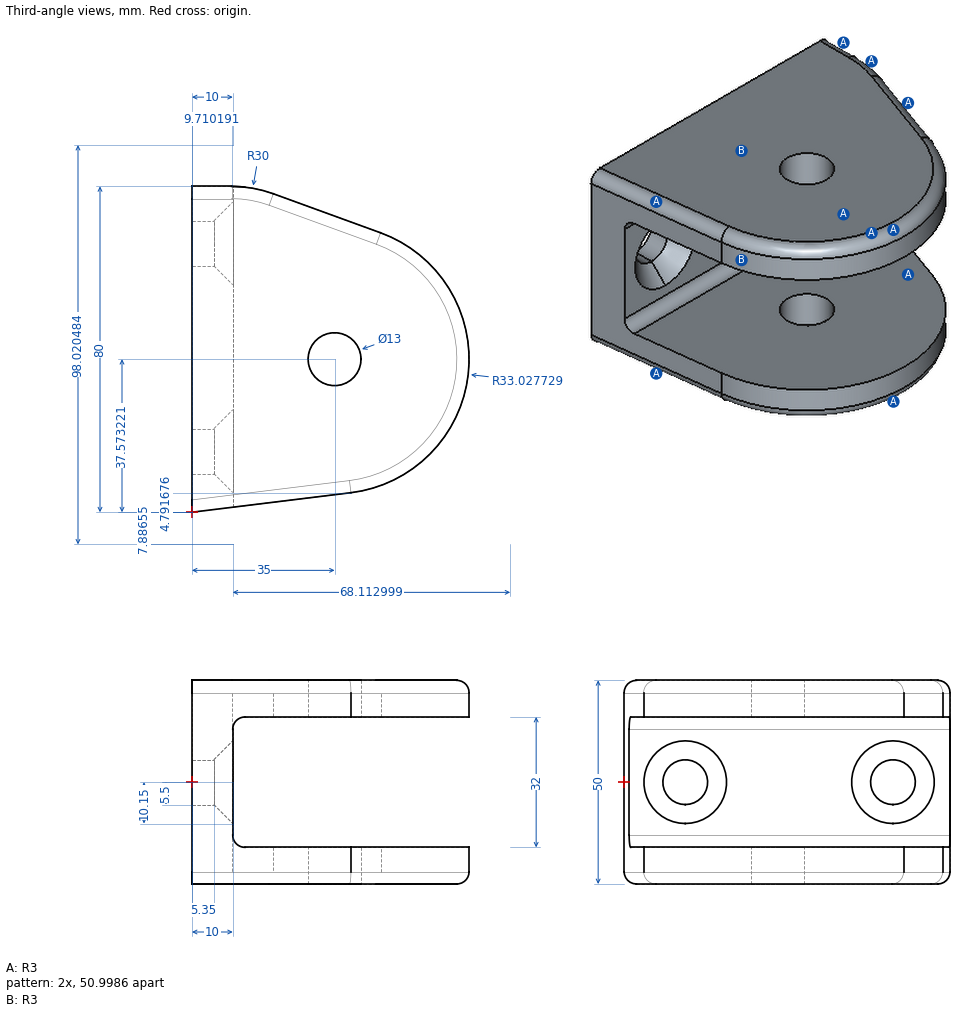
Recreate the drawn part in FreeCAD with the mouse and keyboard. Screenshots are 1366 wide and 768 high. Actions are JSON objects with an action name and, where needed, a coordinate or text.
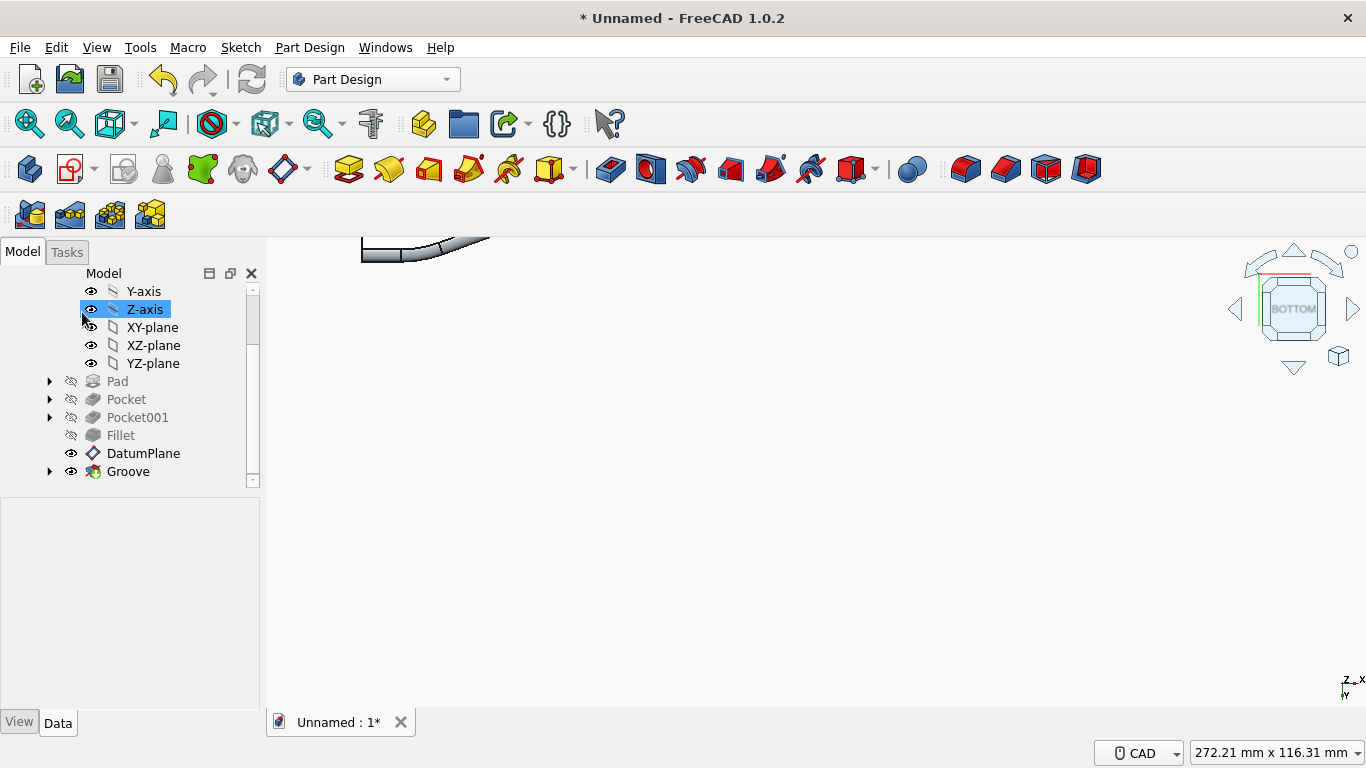
{"action": "left_click", "coordinate": [116, 453]}
{"action": "key", "text": "space"}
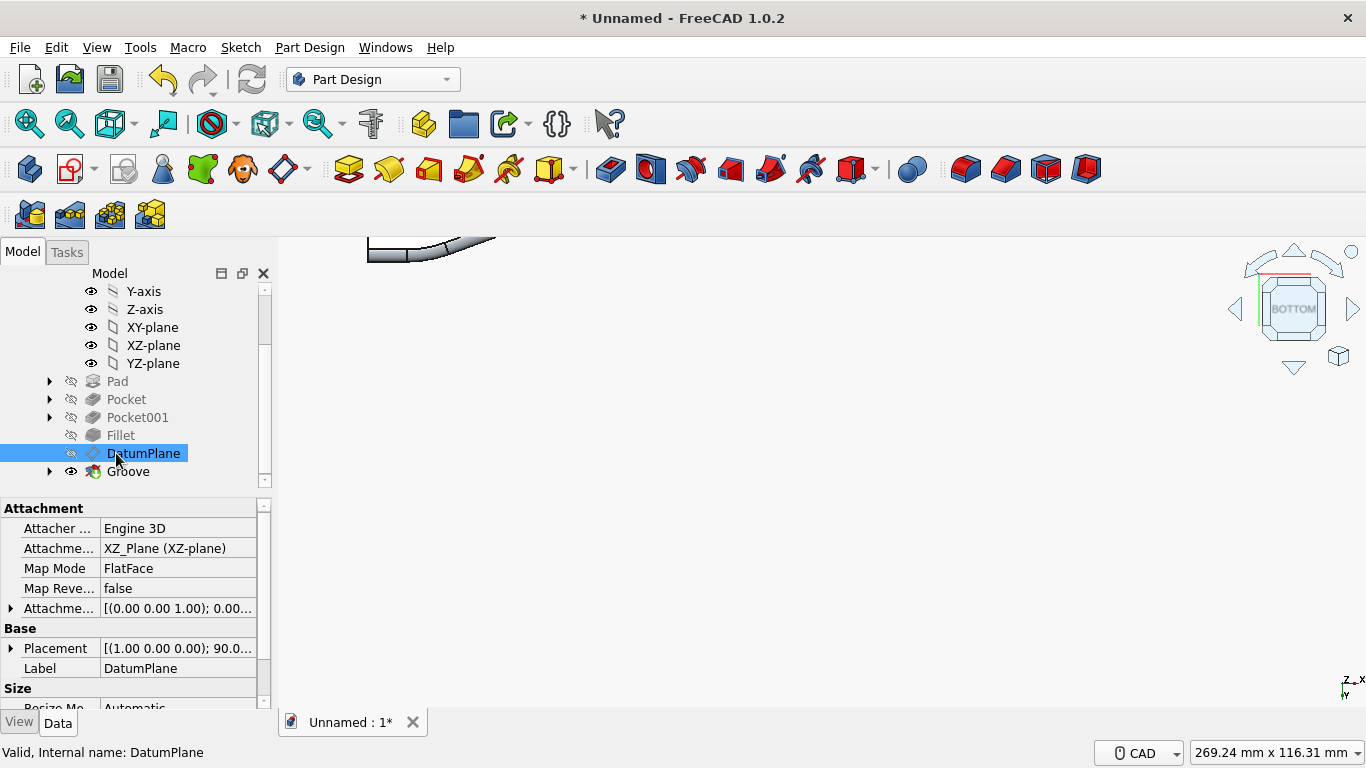
{"action": "left_click", "coordinate": [30, 124]}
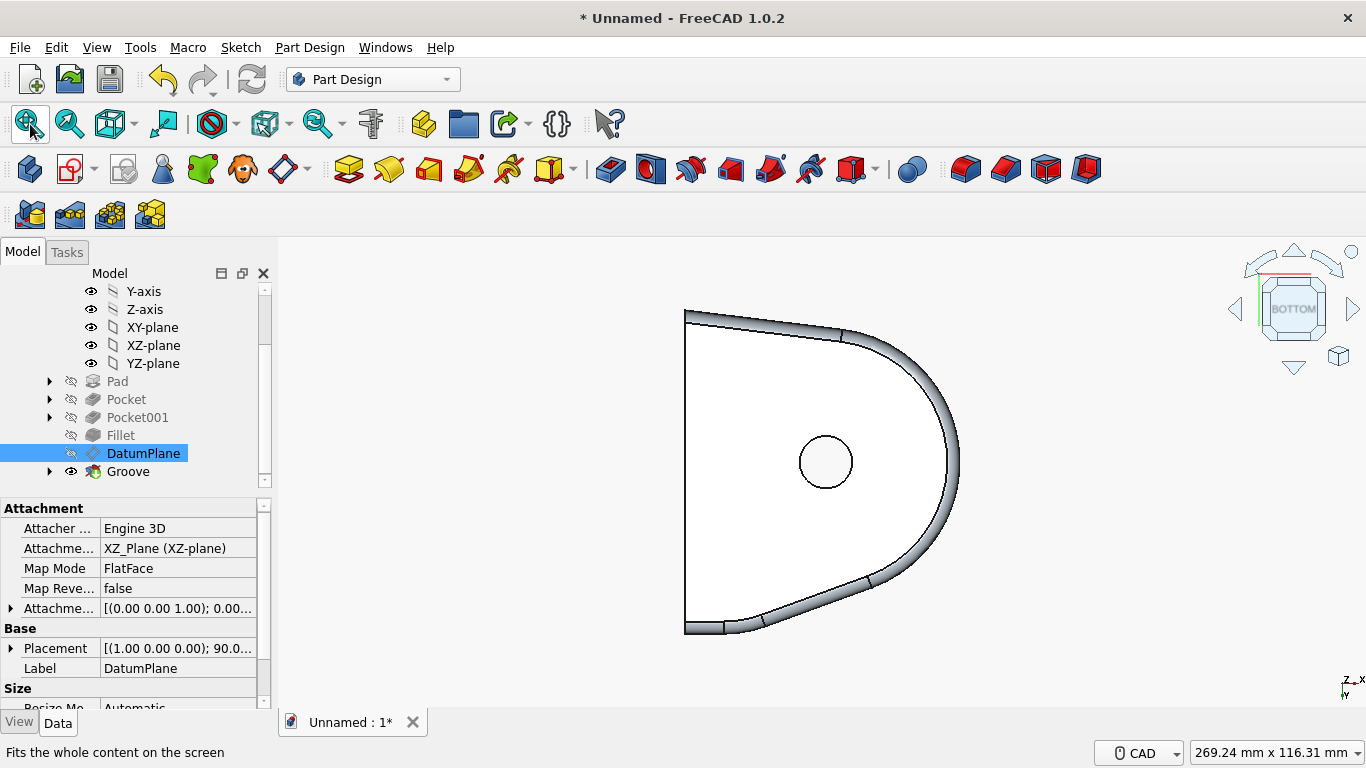
{"action": "left_click", "coordinate": [116, 471]}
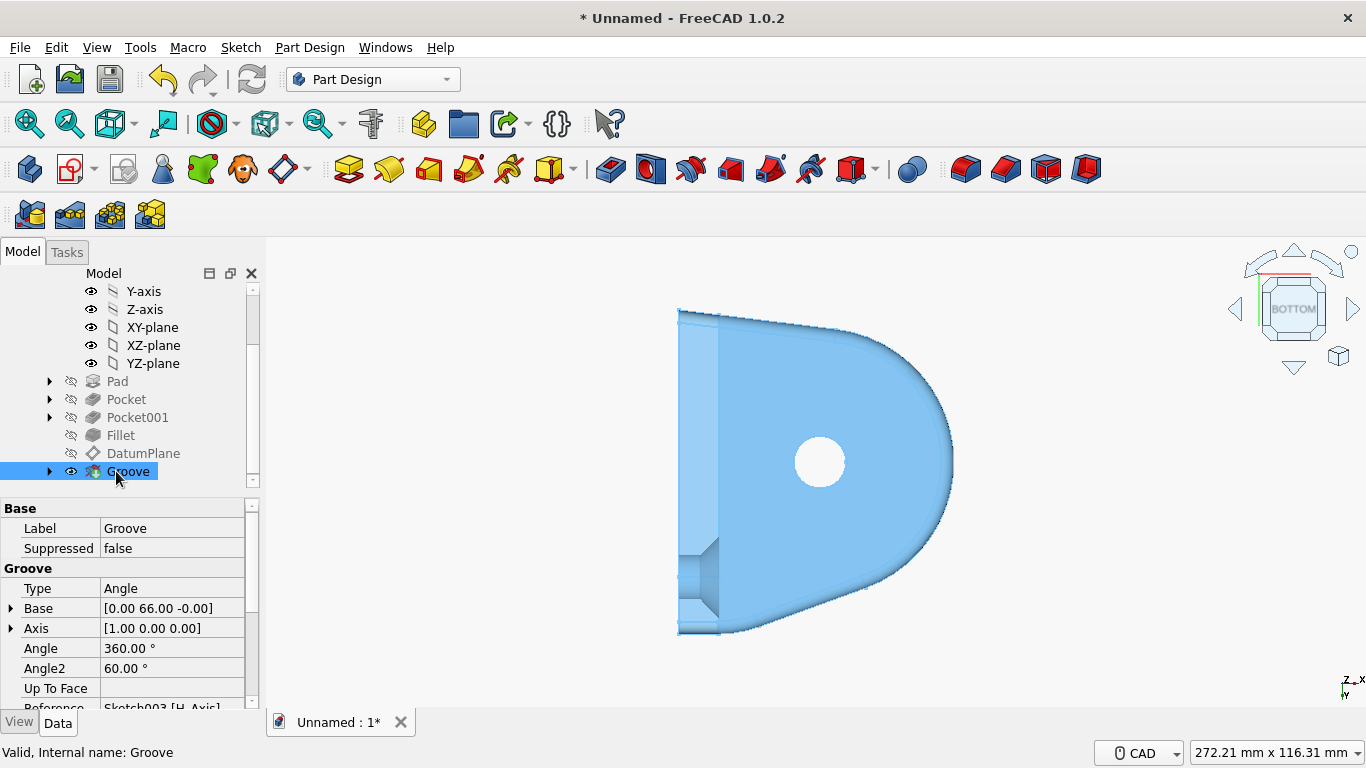
{"action": "left_click", "coordinate": [70, 214]}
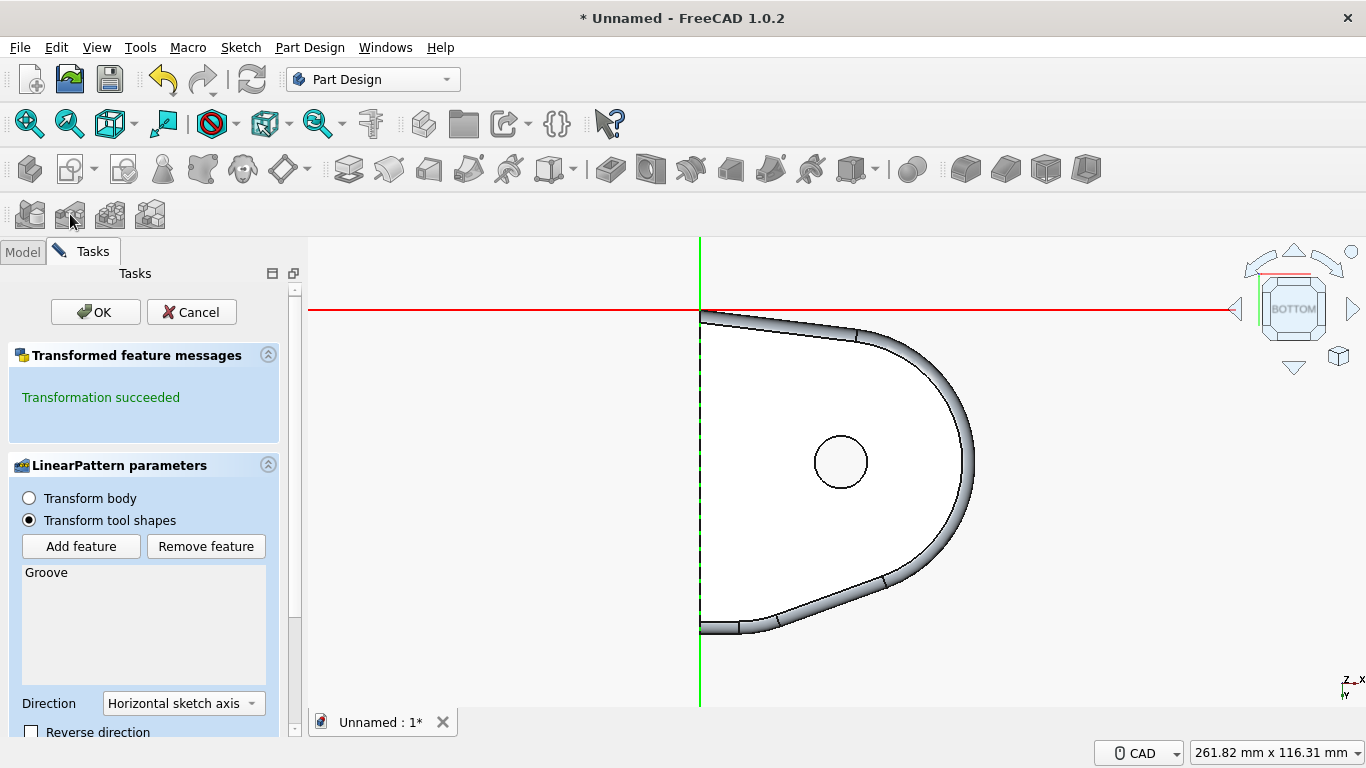
{"action": "left_click", "coordinate": [184, 704]}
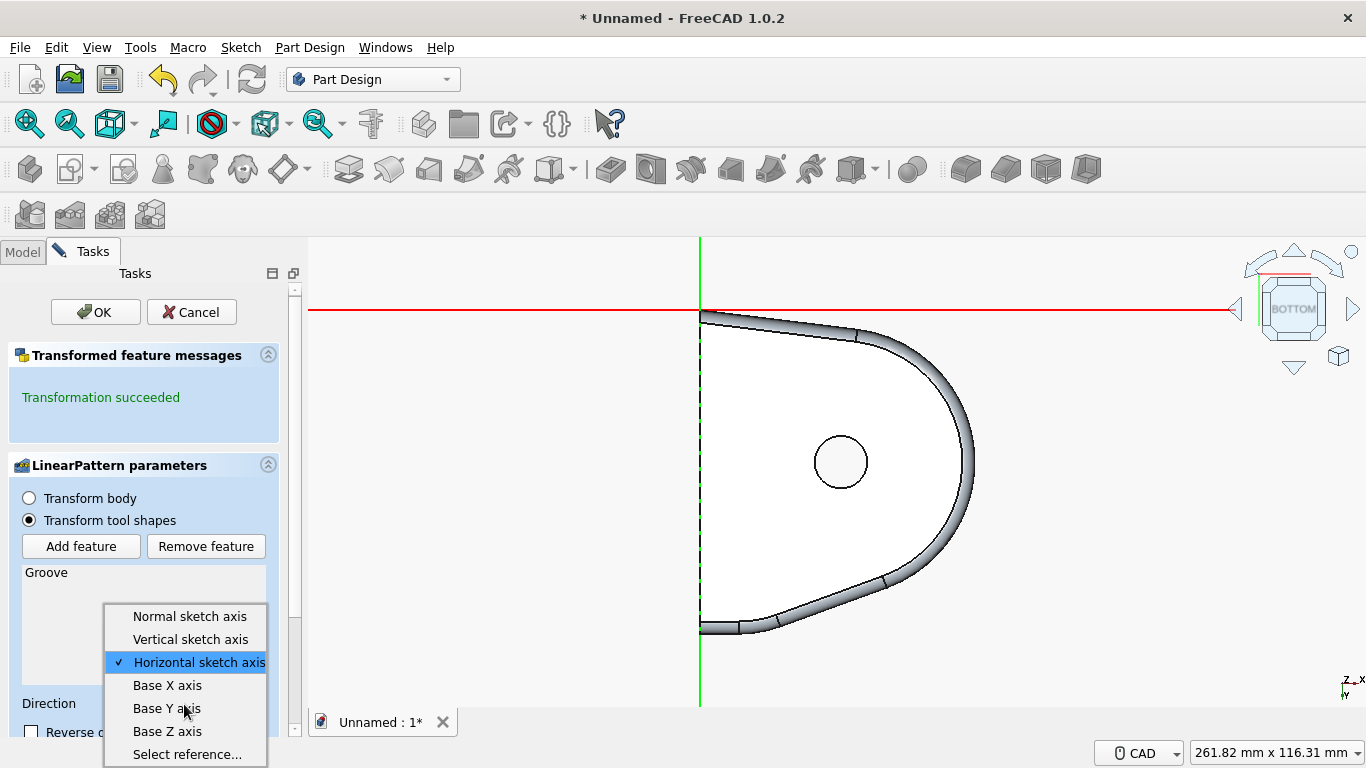
{"action": "left_click", "coordinate": [184, 708]}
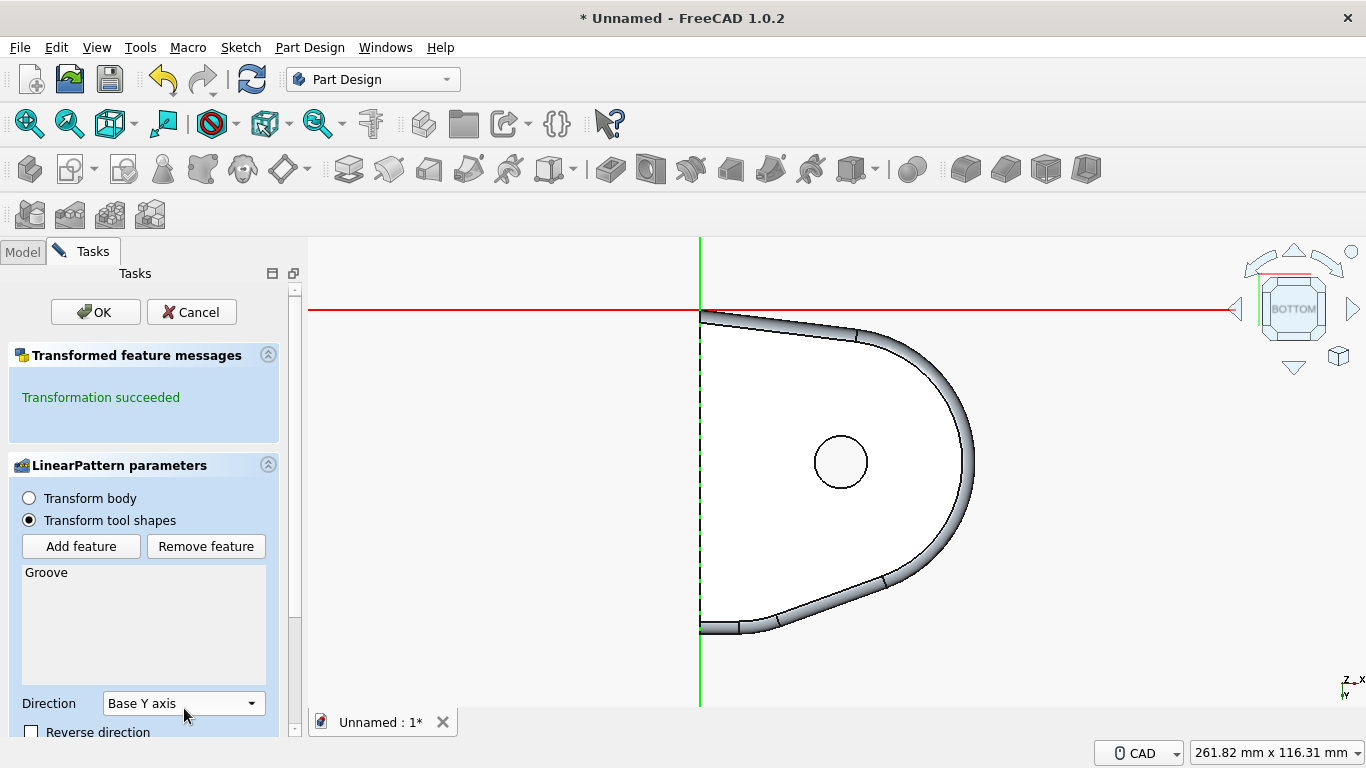
{"action": "scroll", "coordinate": [295, 510], "scroll_direction": "down", "scroll_amount": 2}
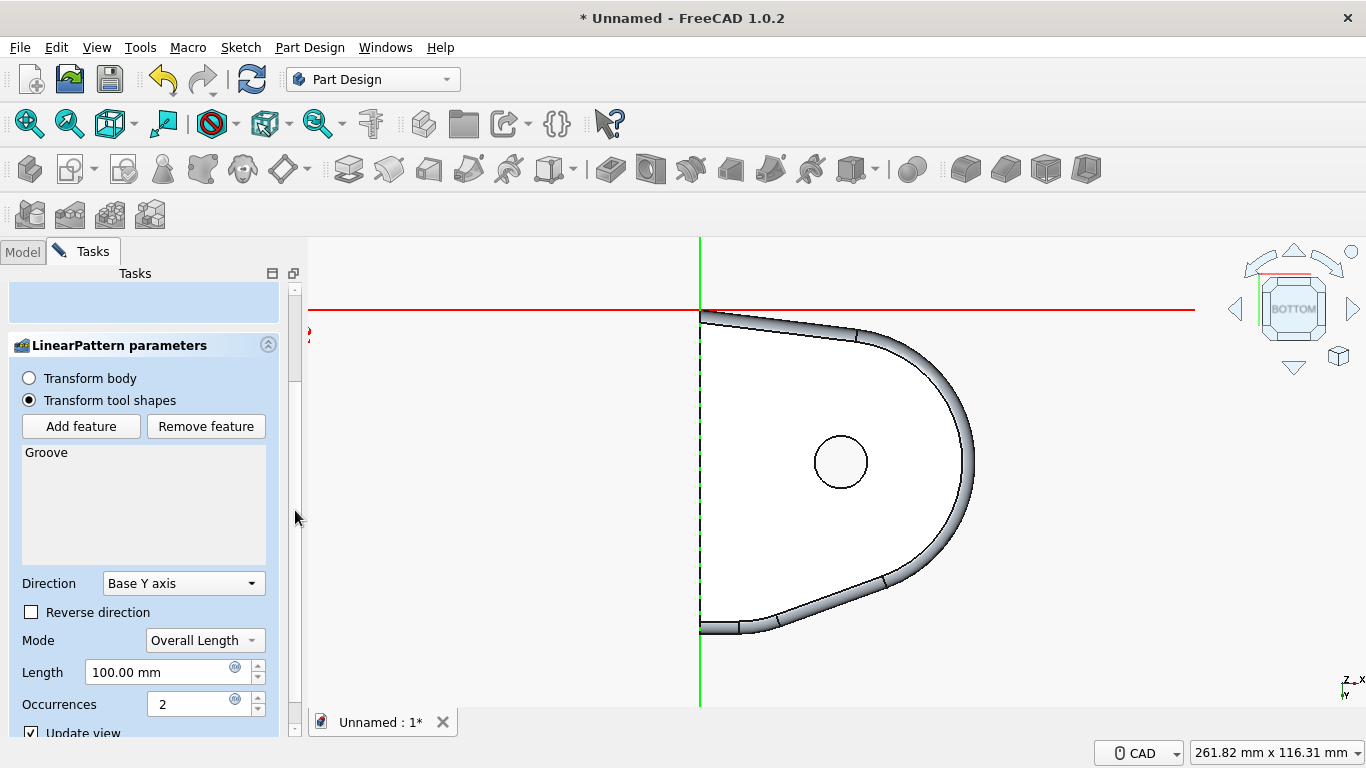
{"action": "left_click", "coordinate": [206, 640]}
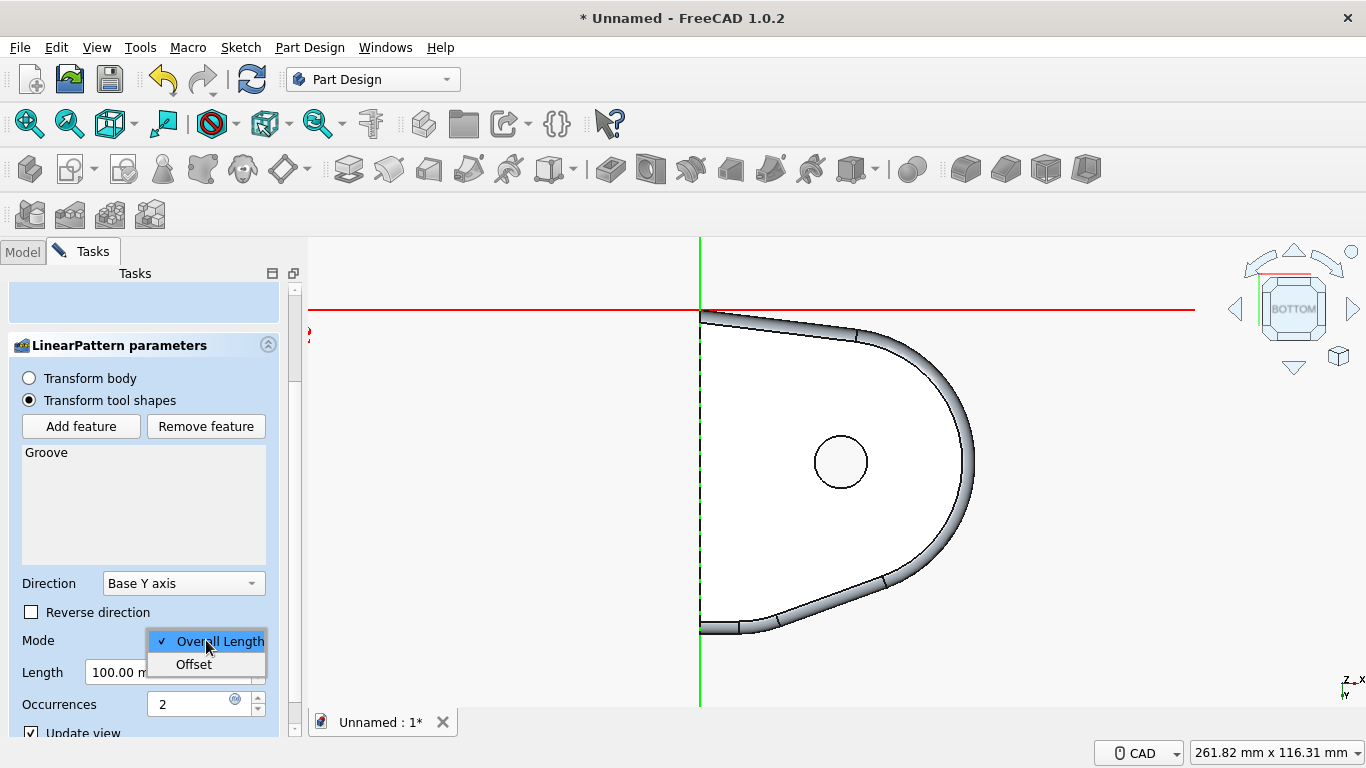
{"action": "left_click", "coordinate": [206, 664]}